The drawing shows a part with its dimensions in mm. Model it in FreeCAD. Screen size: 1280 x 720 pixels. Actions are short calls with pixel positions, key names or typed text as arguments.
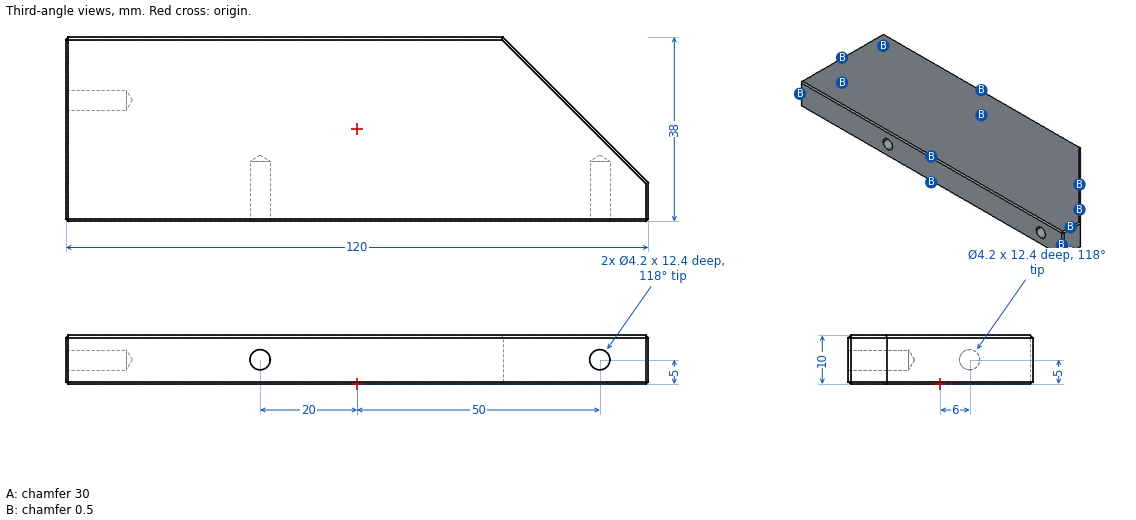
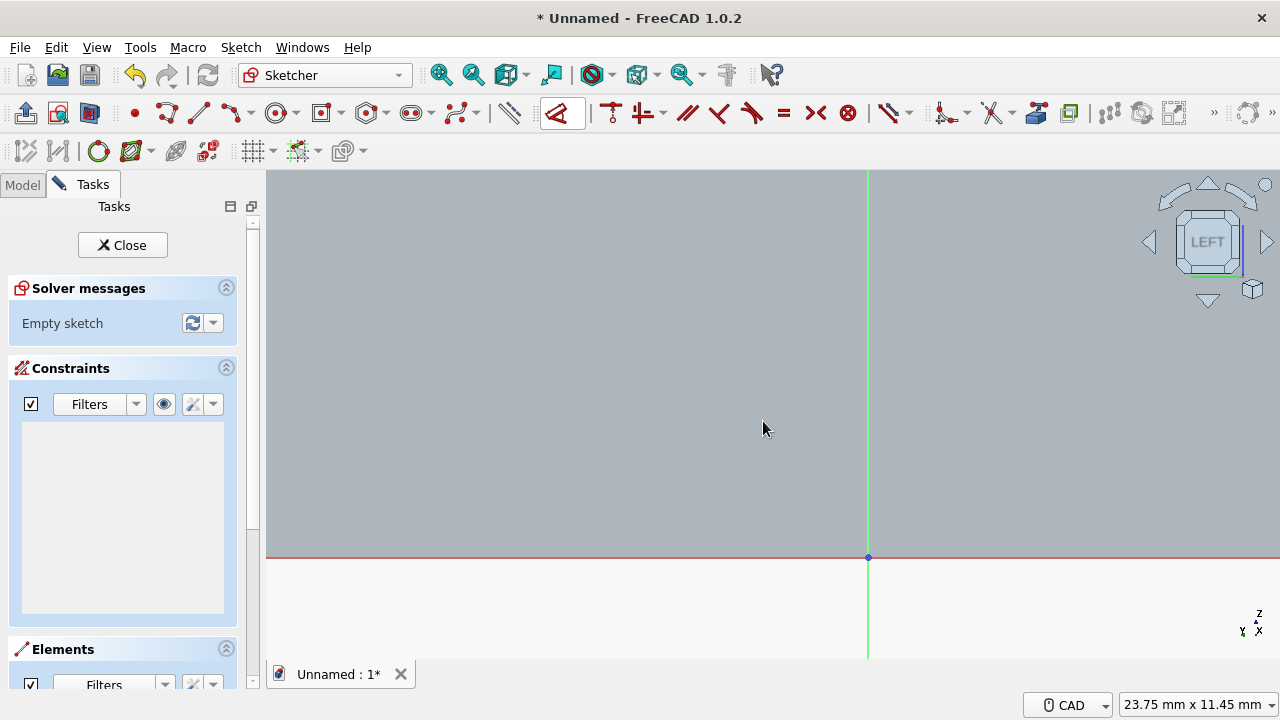
click(276, 114)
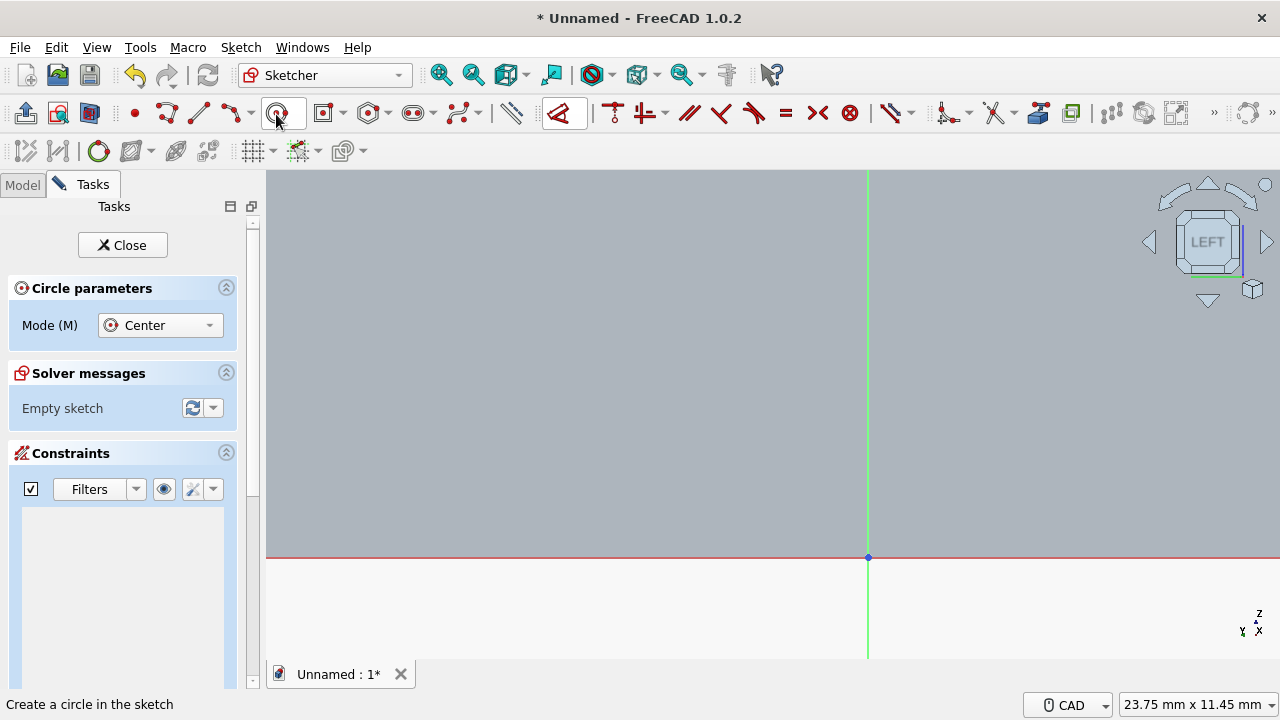
click(612, 344)
click(676, 281)
key(Escape)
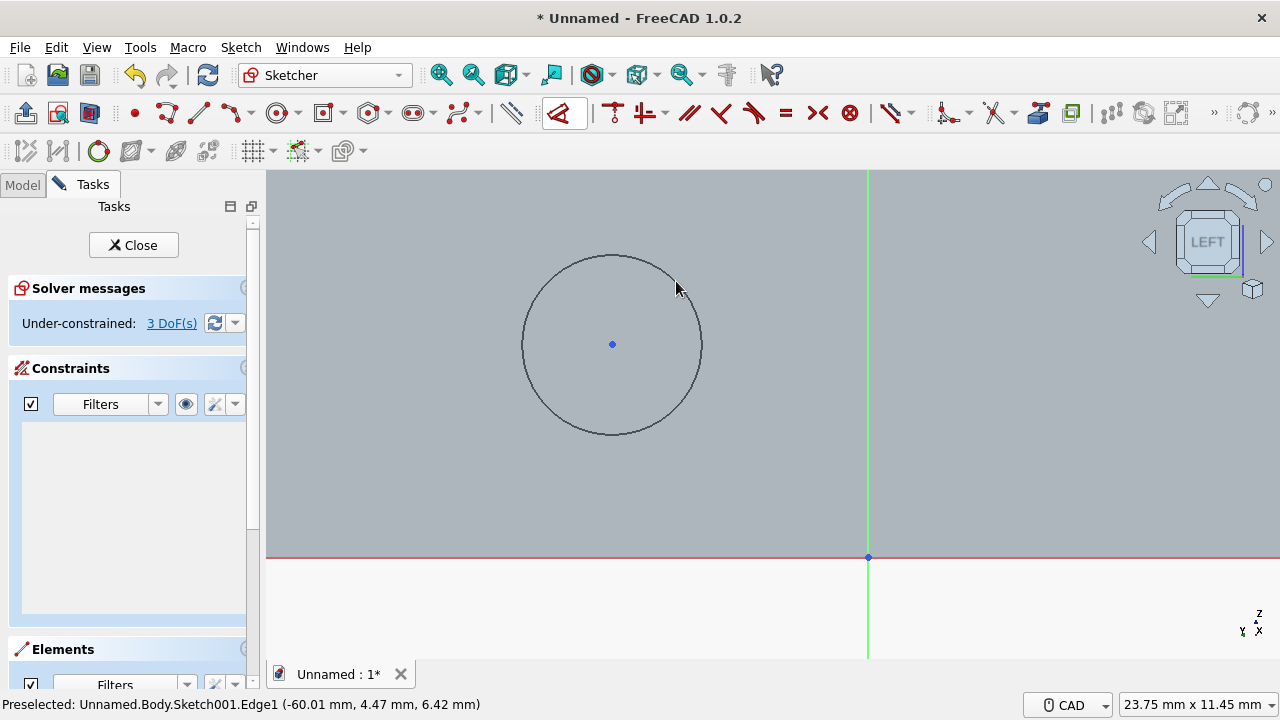
click(675, 281)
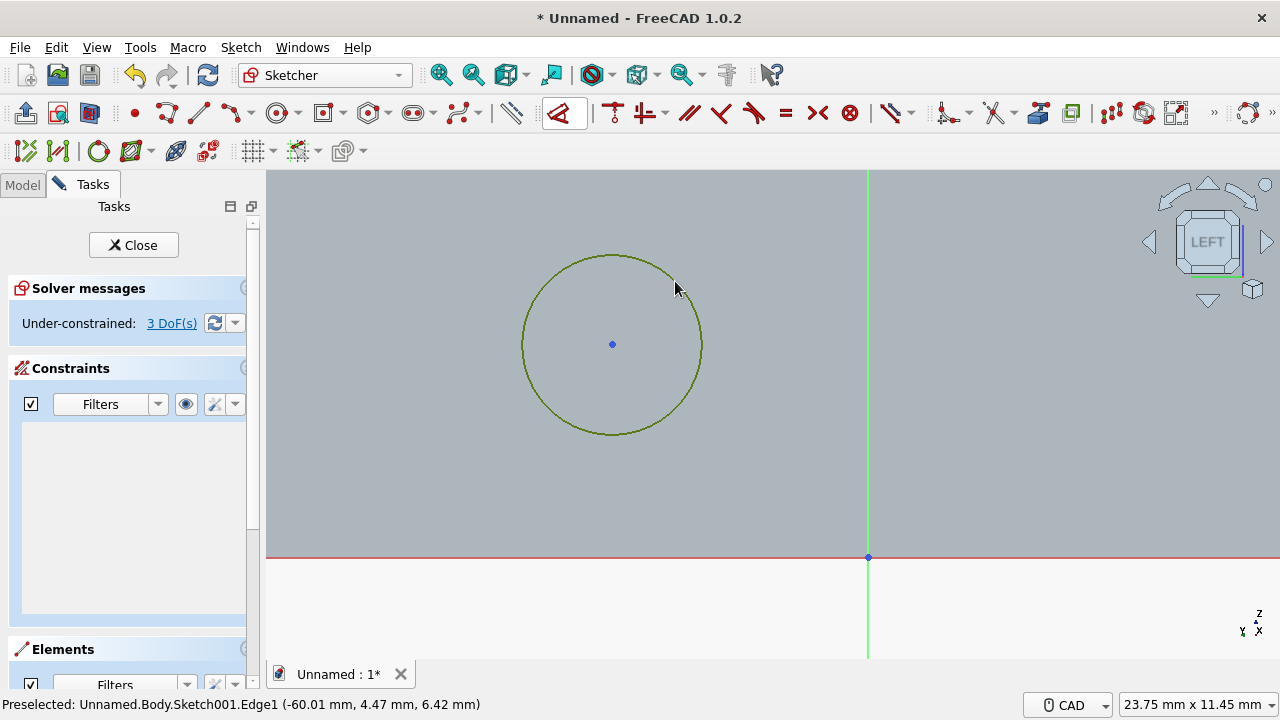
key(k)
key(o)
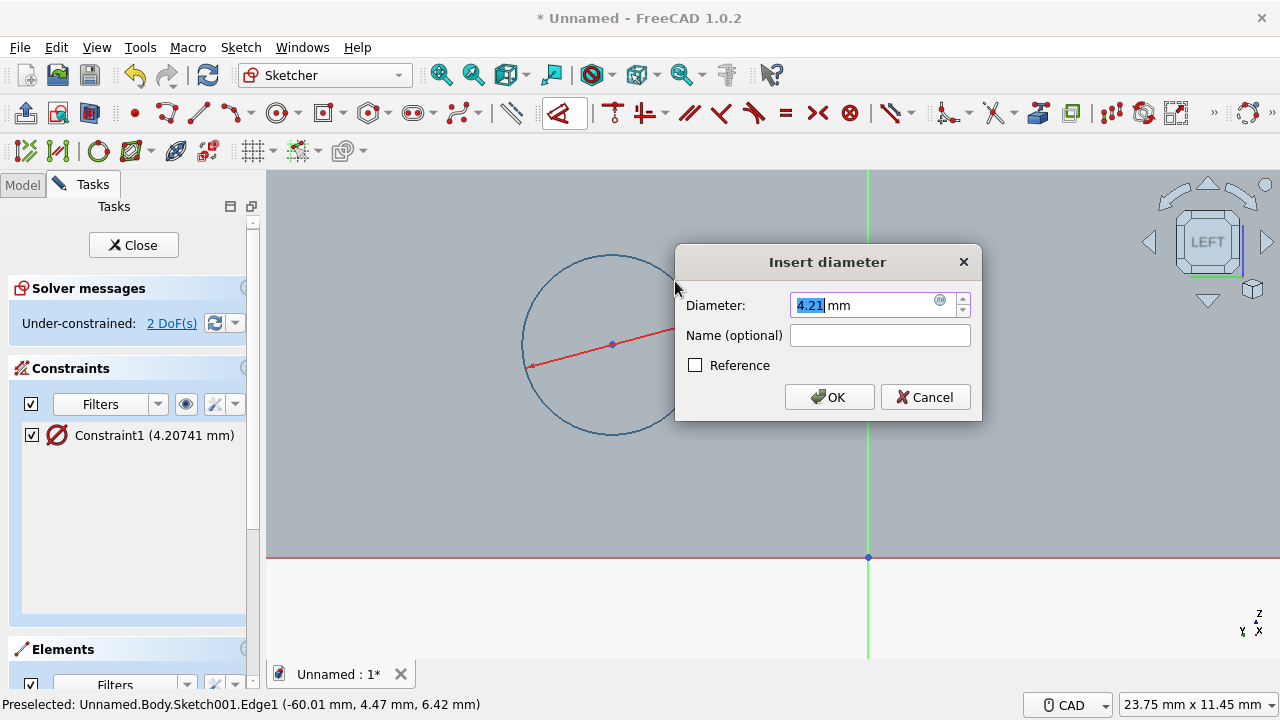
text(4.2)
key(Return)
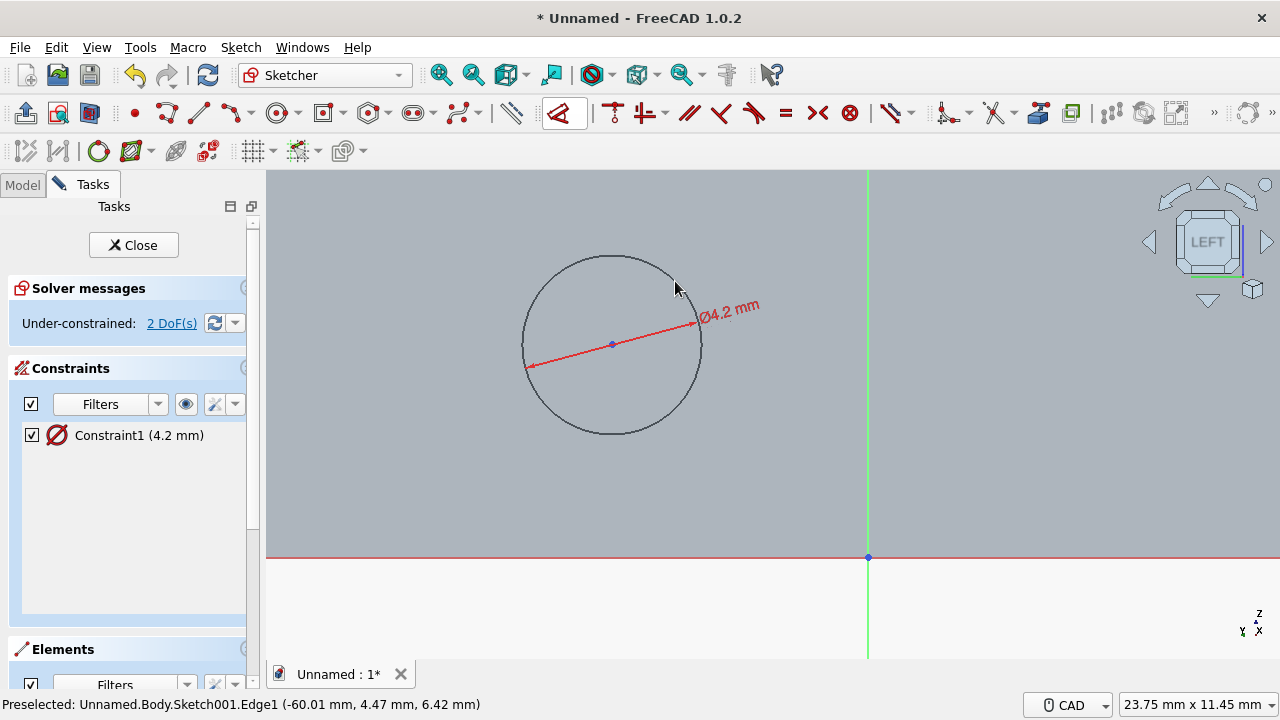
click(612, 345)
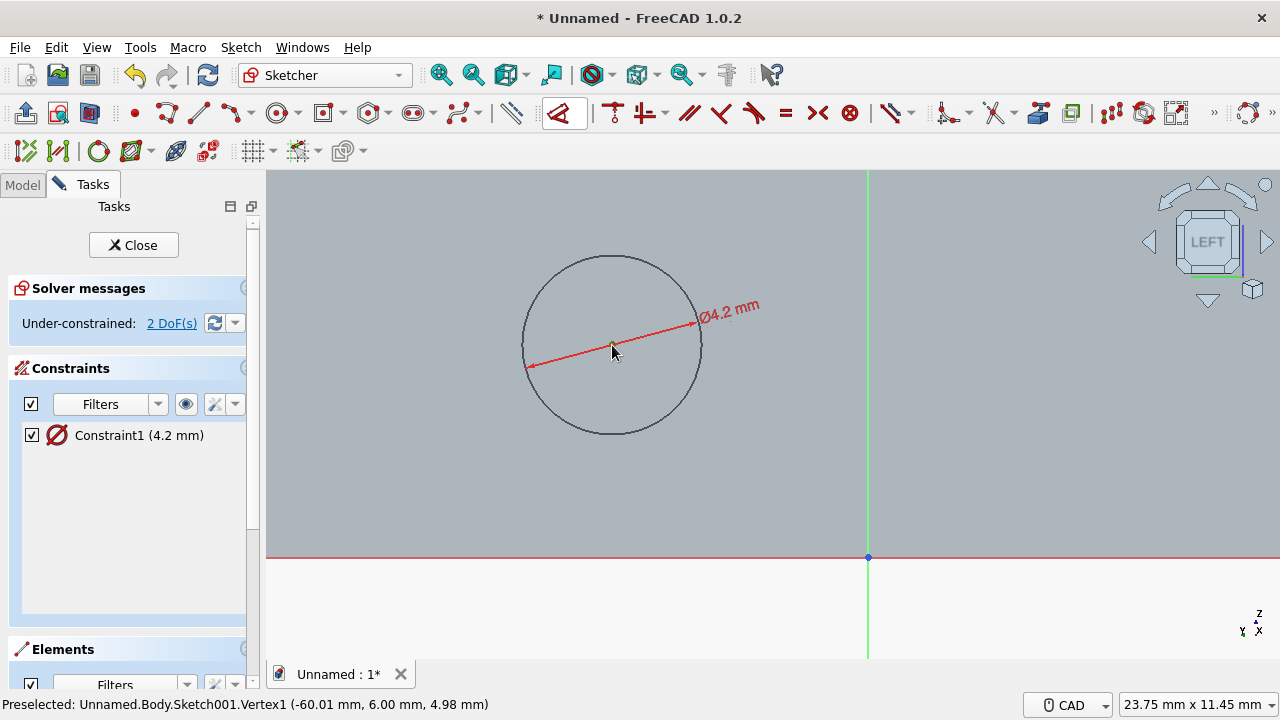
click(582, 114)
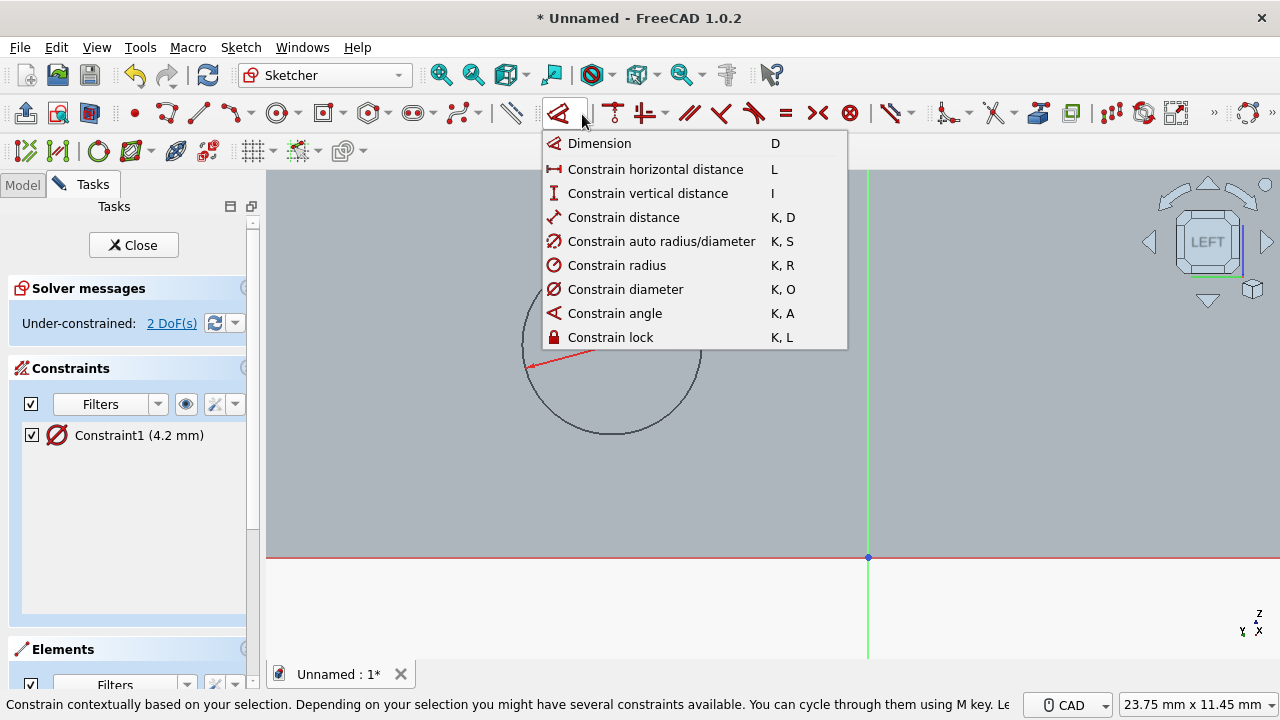
click(695, 169)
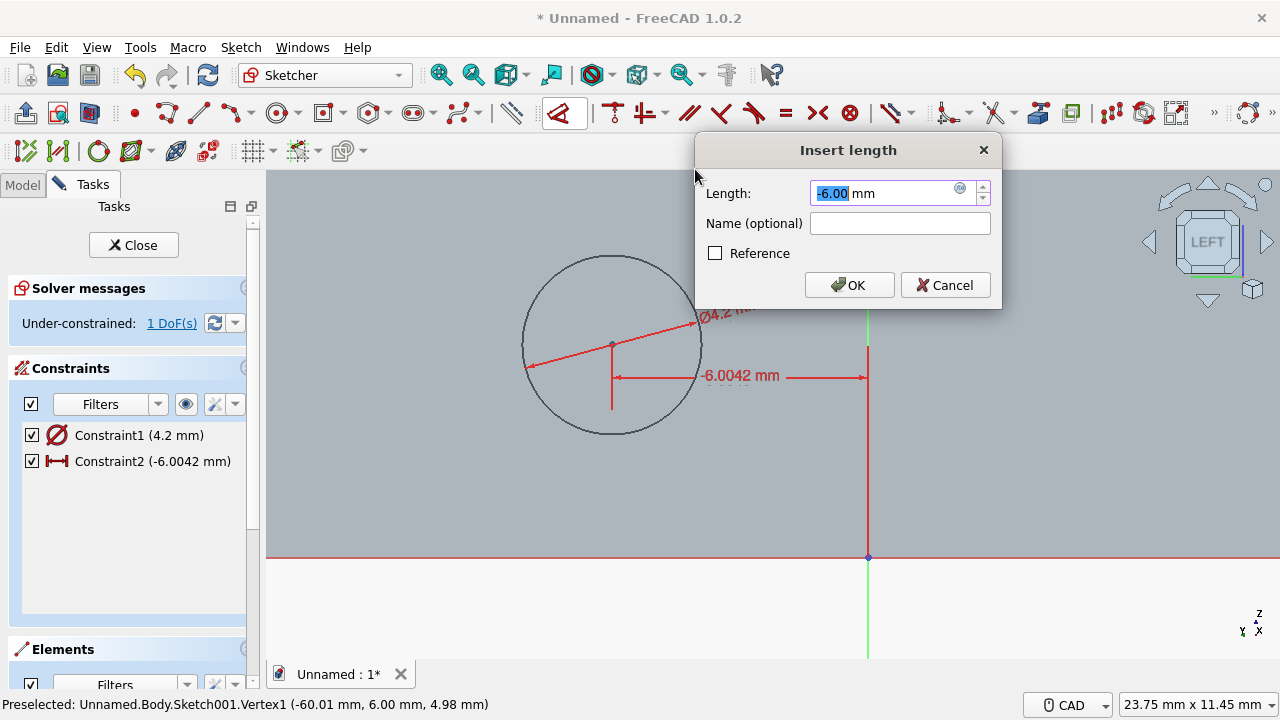
text(-6)
key(Return)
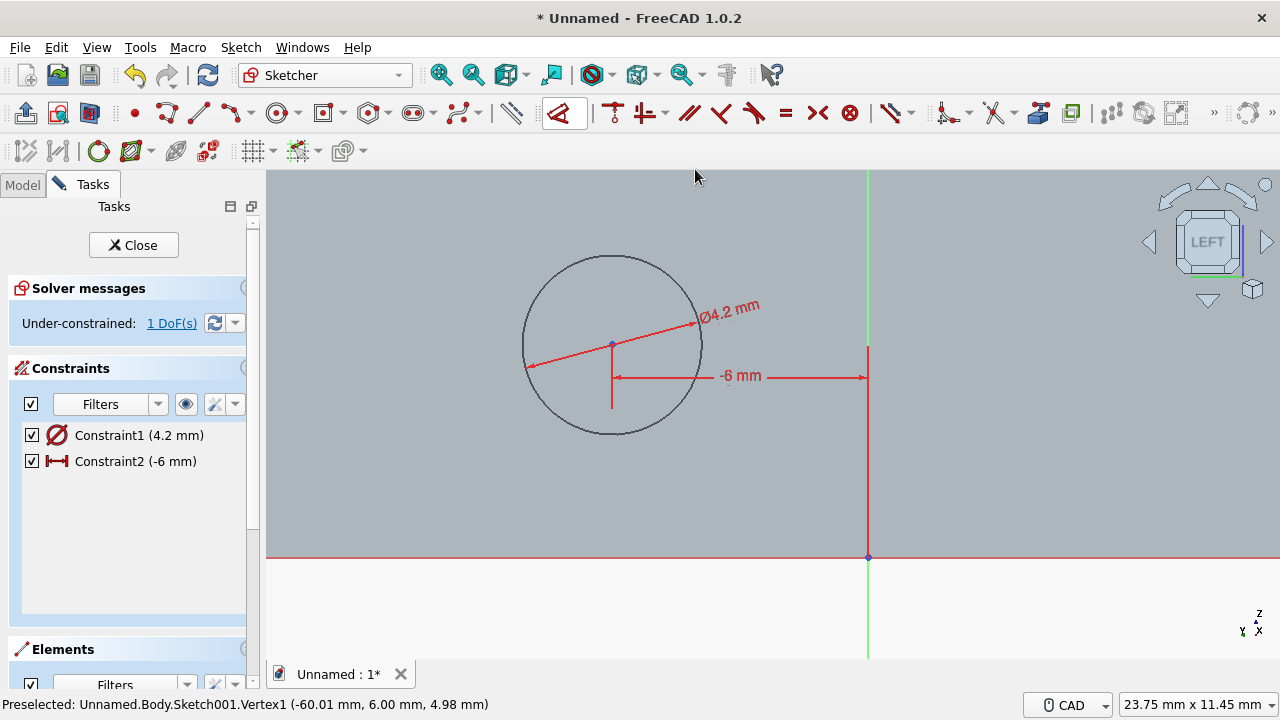
click(612, 345)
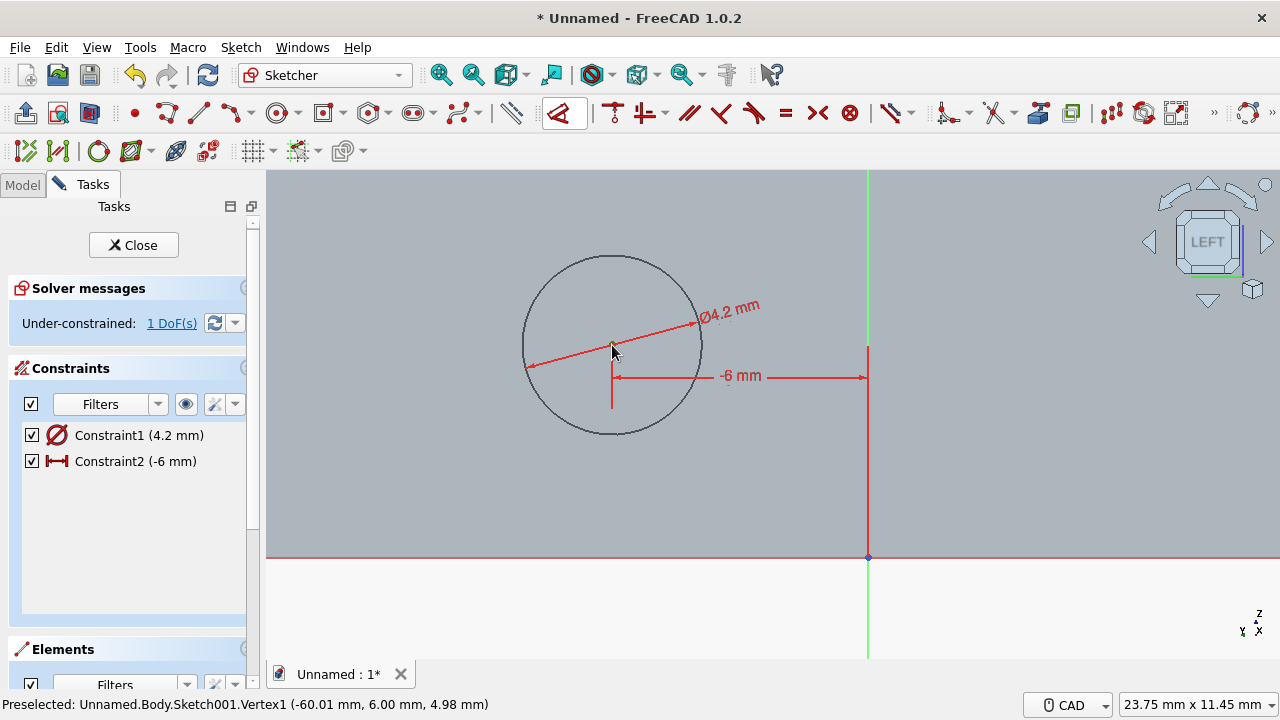
click(582, 114)